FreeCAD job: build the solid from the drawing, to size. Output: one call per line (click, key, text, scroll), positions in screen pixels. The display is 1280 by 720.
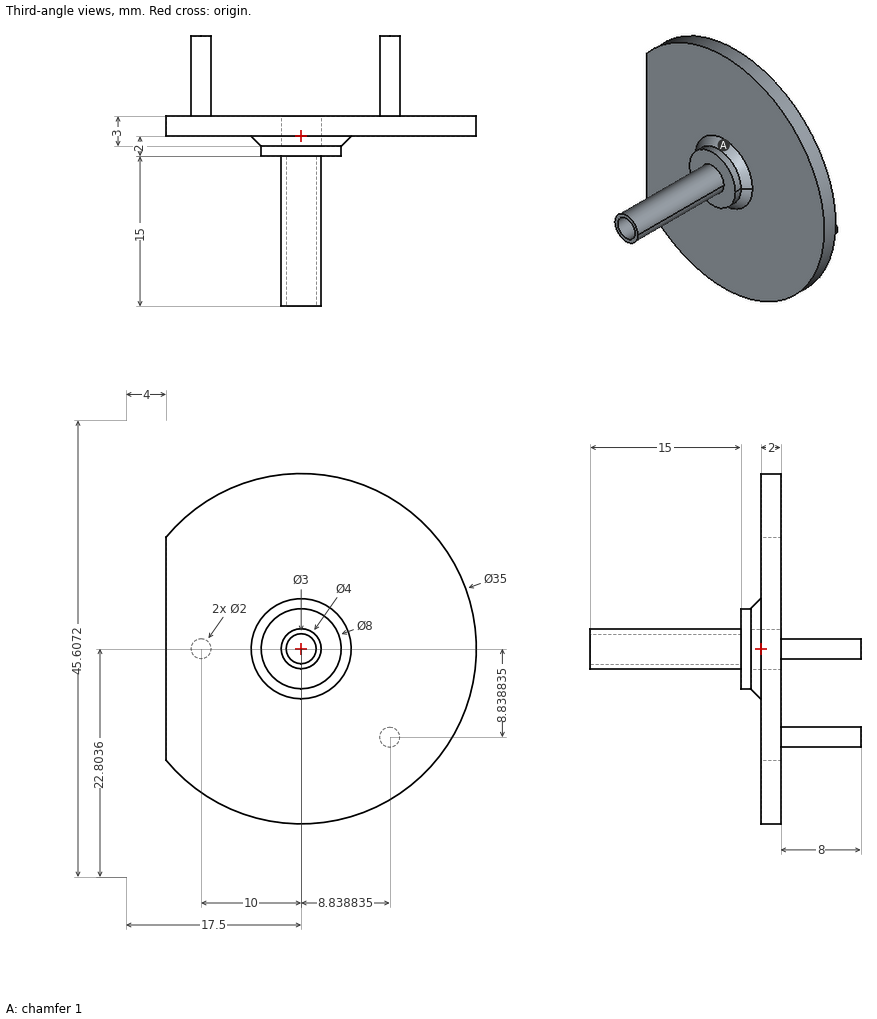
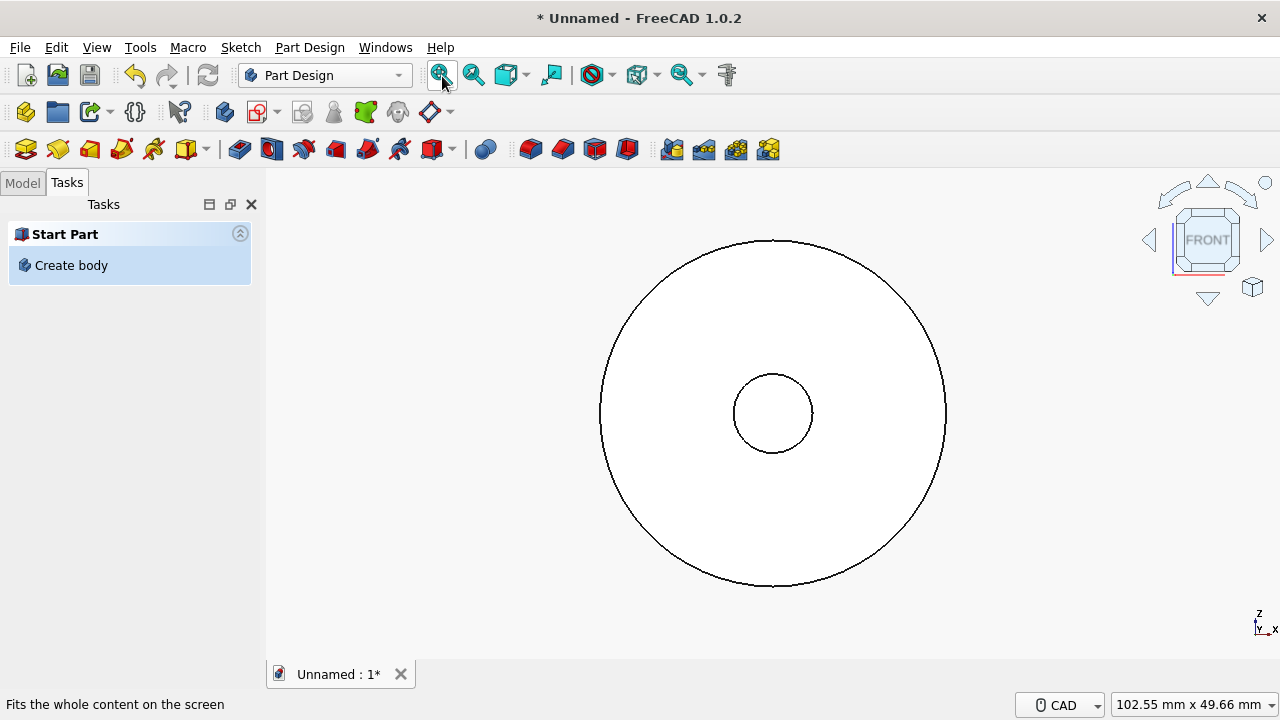
key(3)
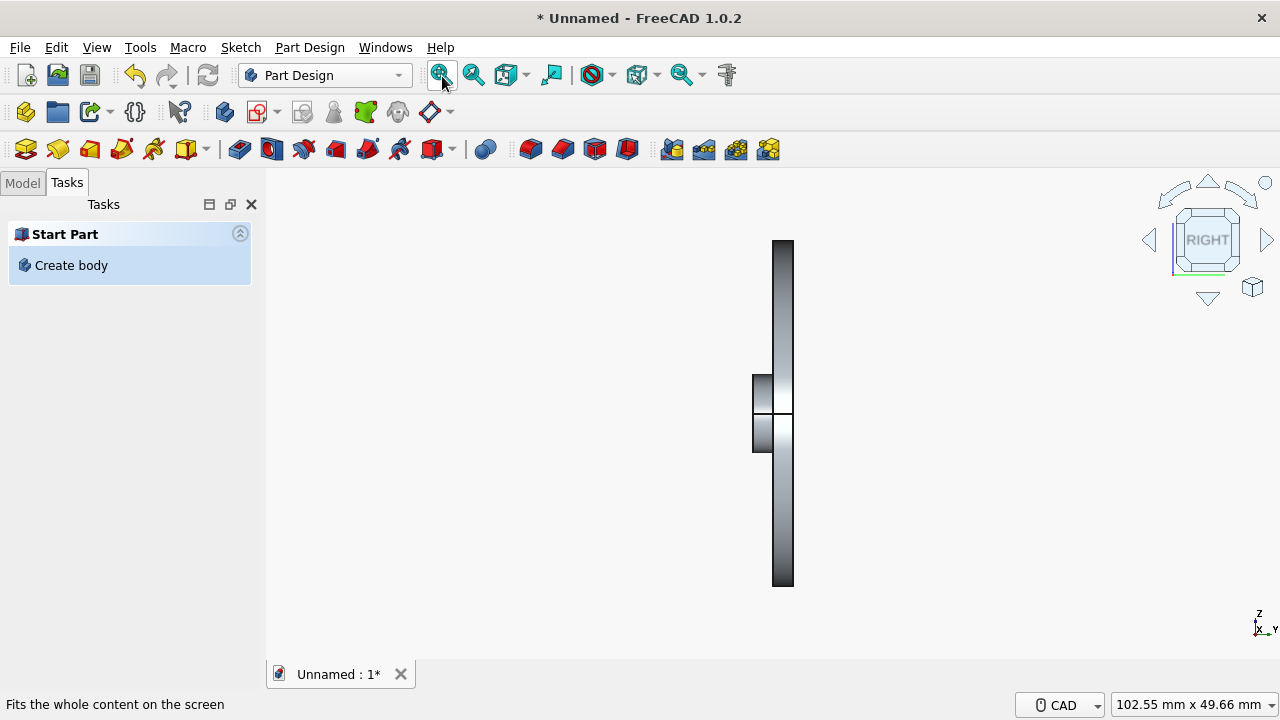
key(5)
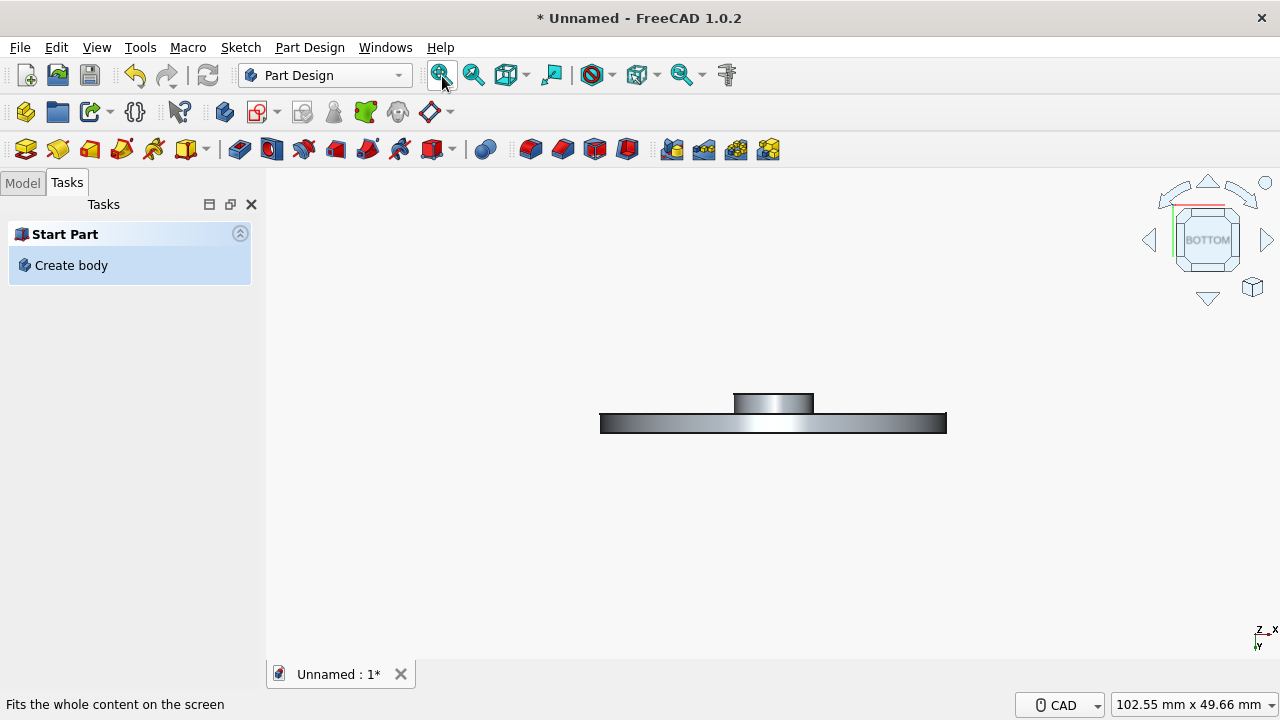
click(442, 76)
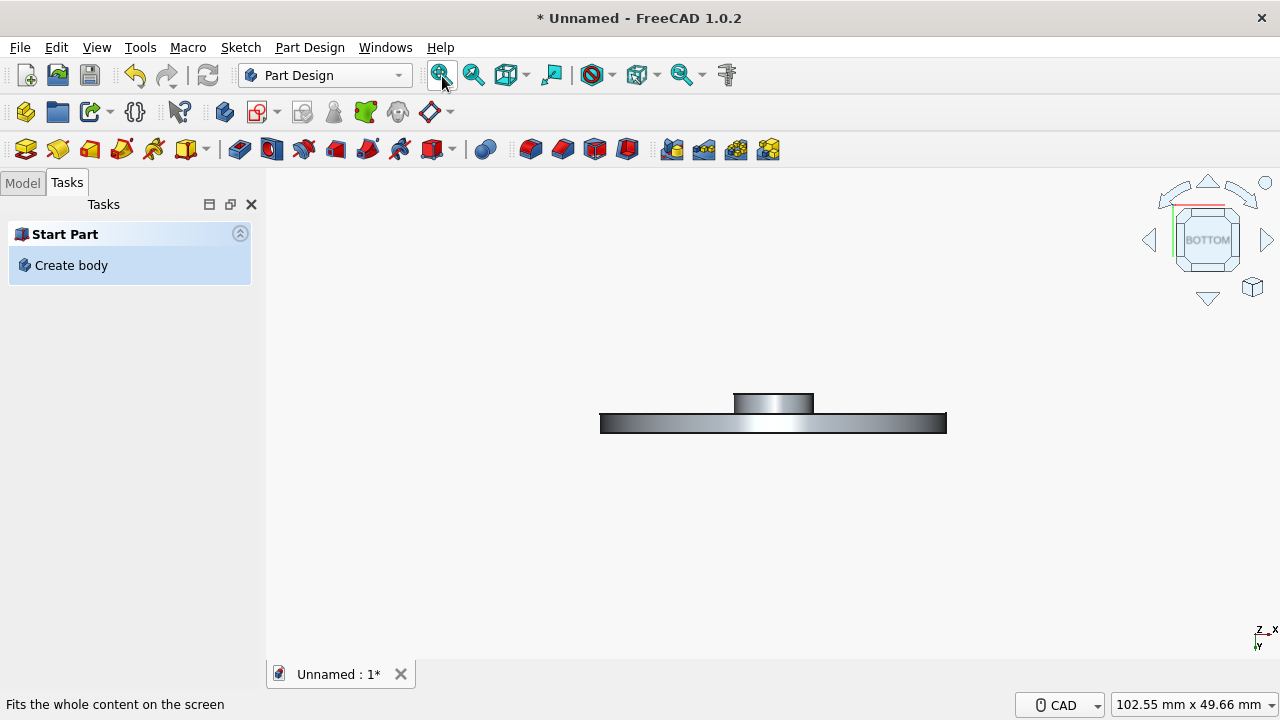
key(4)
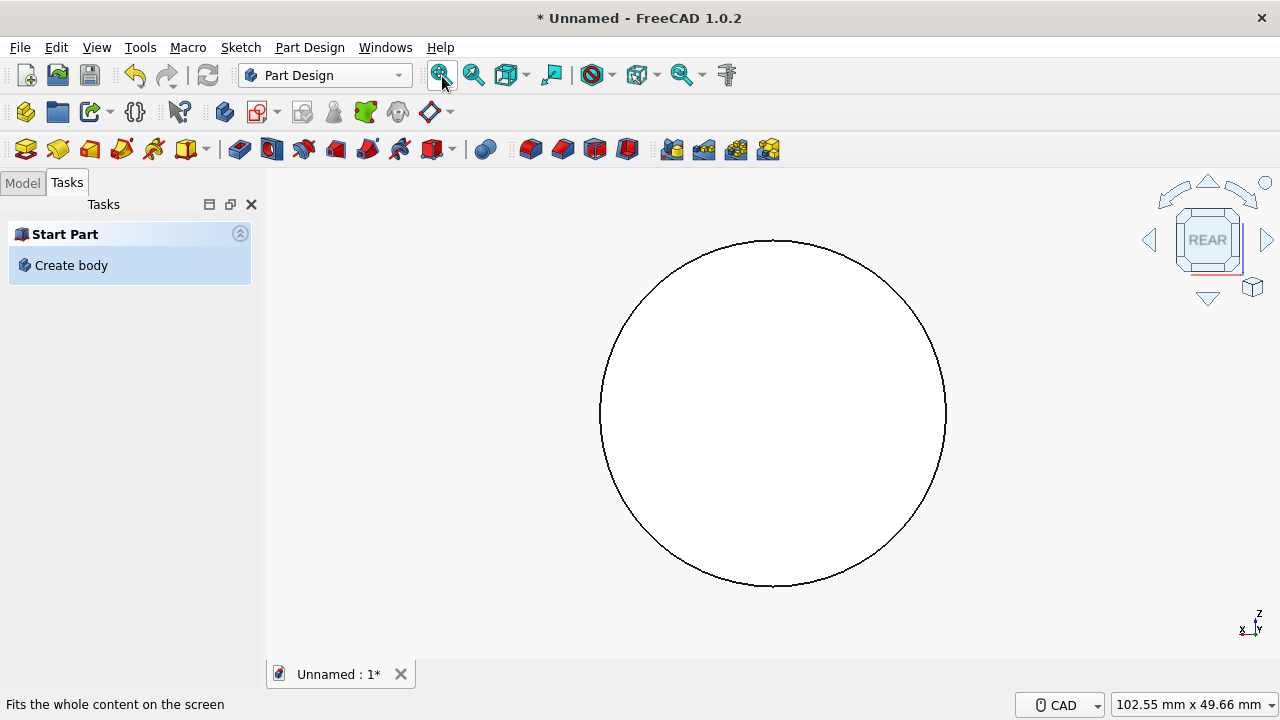
key(6)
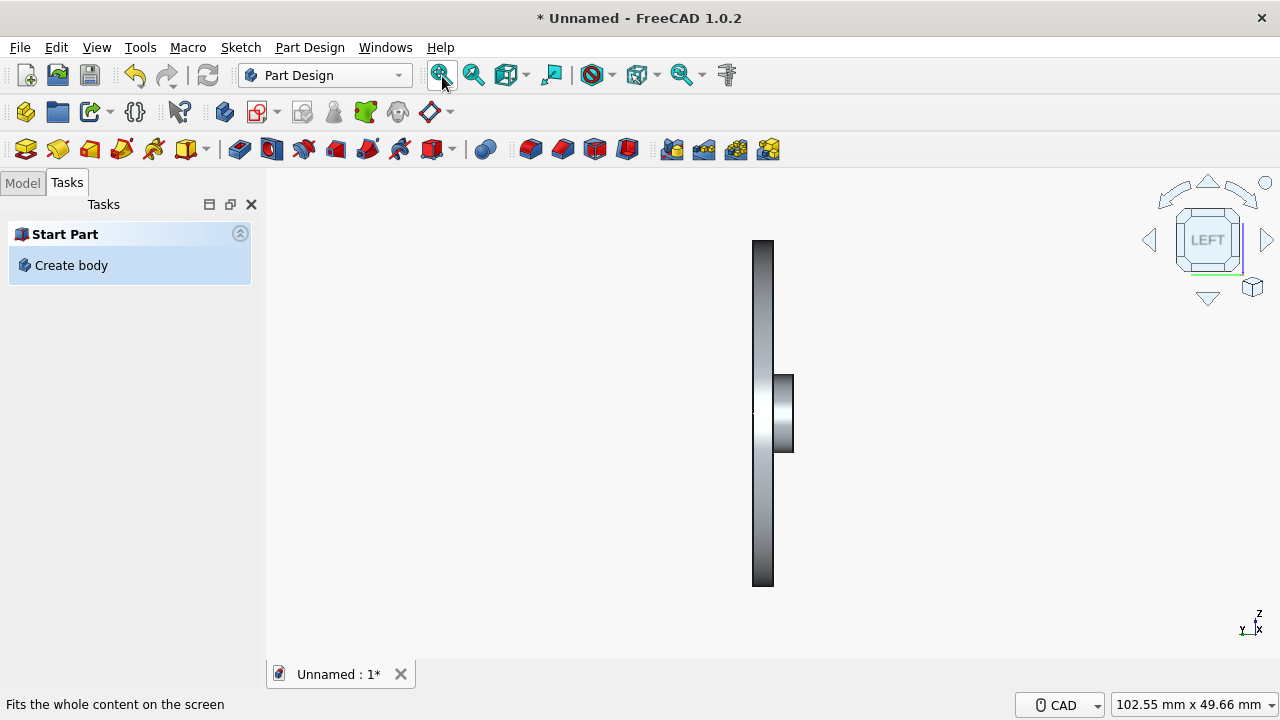
key(v)
key(3)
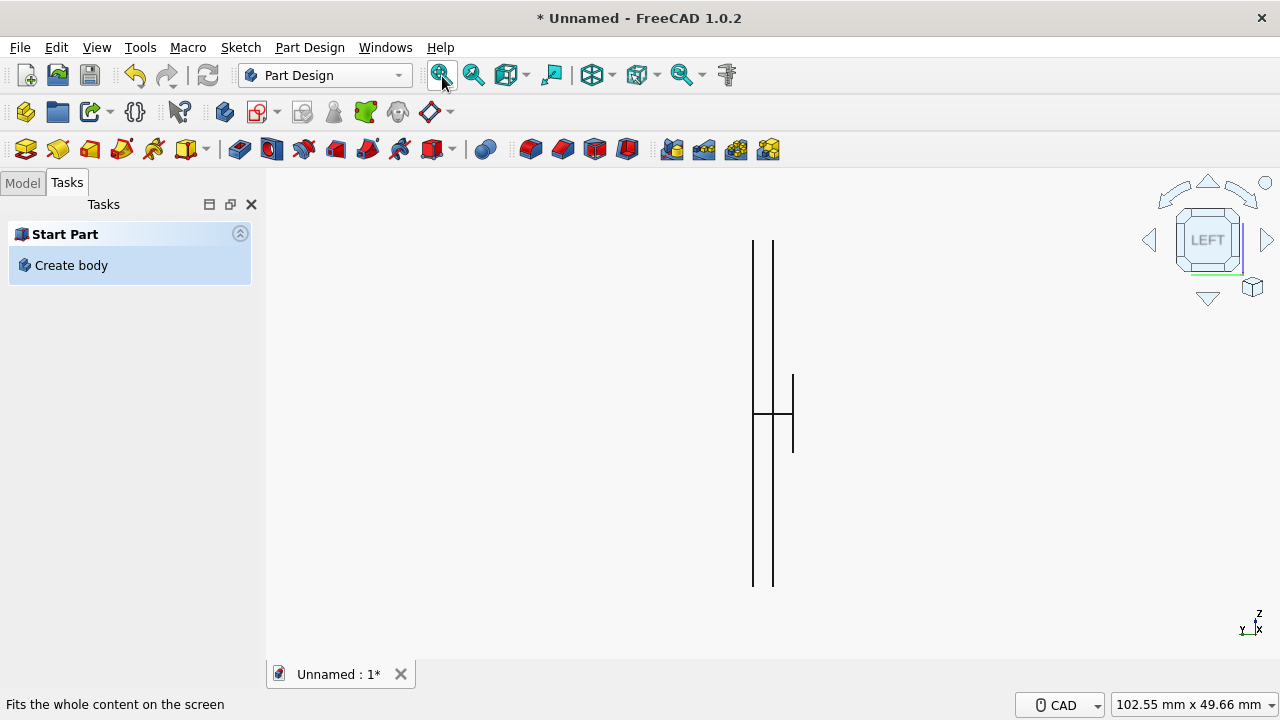
key(0)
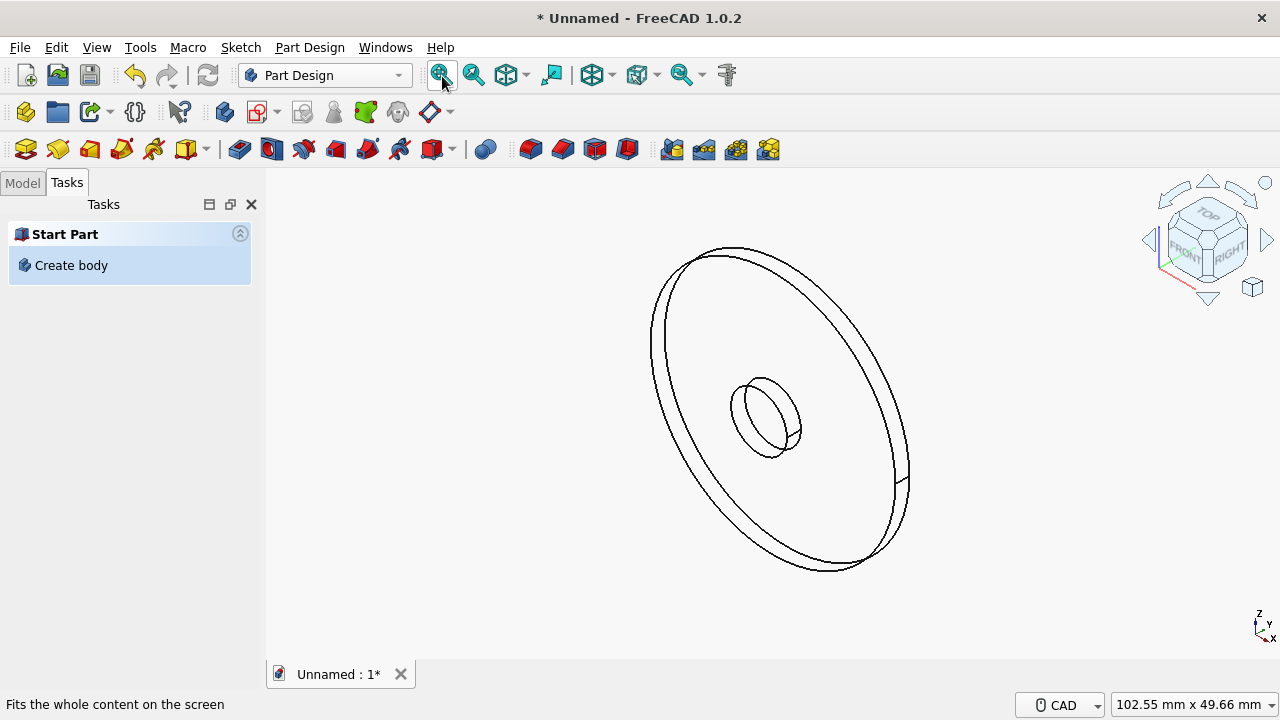
click(745, 396)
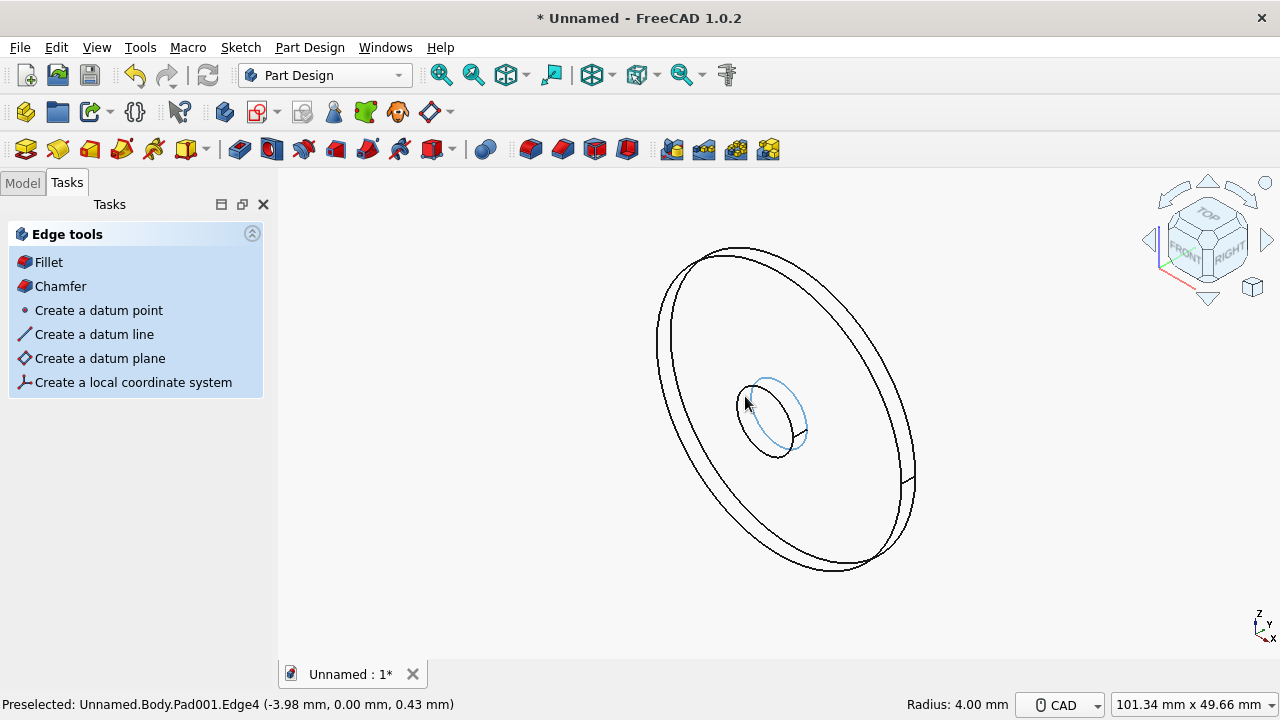
key(v)
key(1)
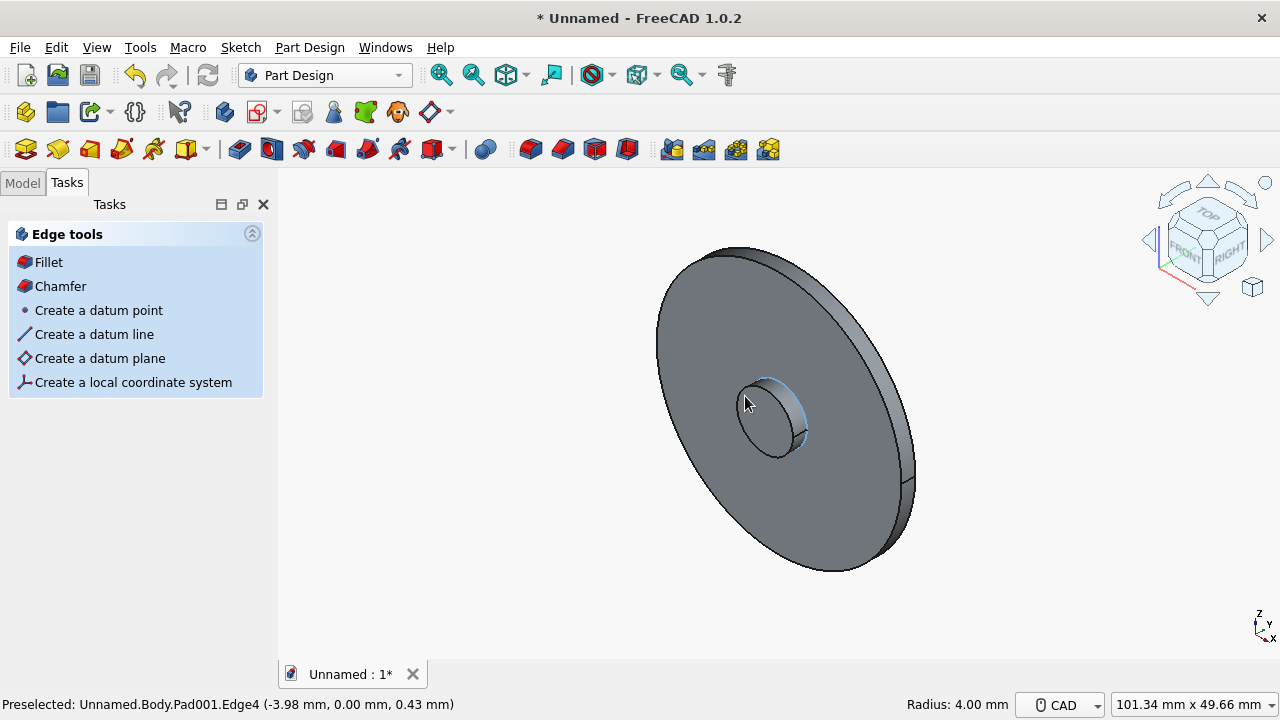
click(564, 150)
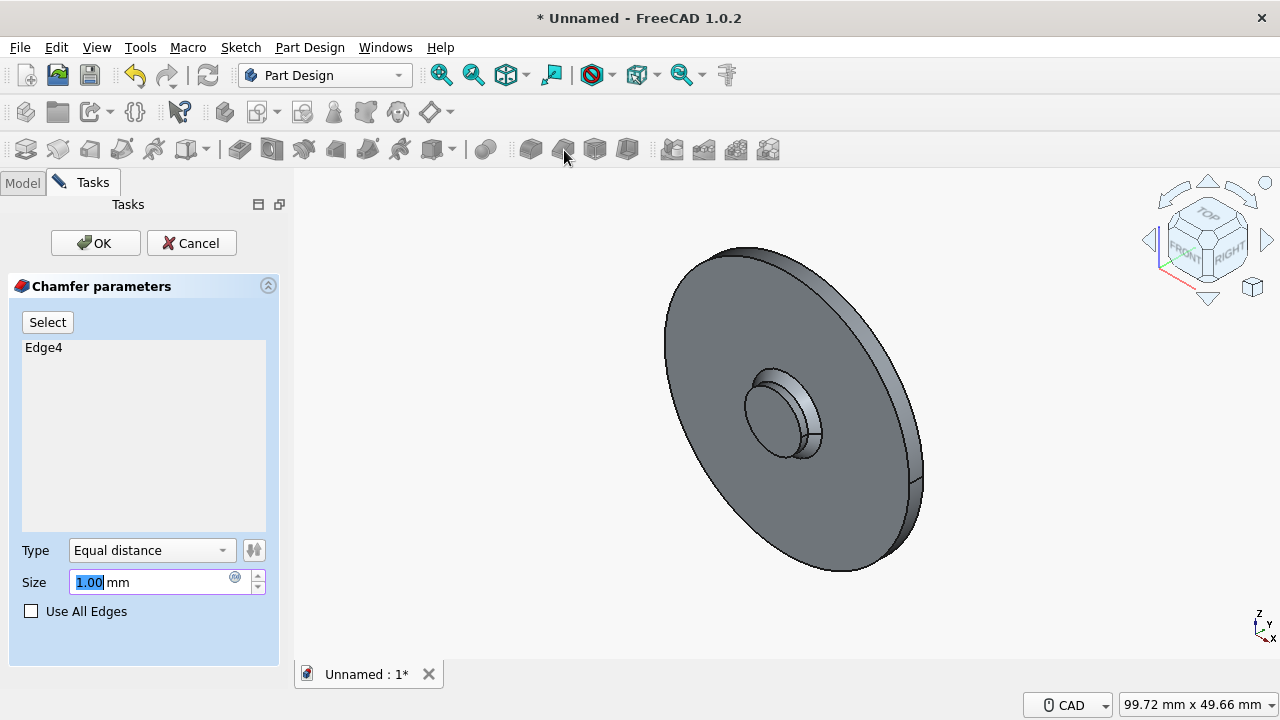
text(1)
key(Tab)